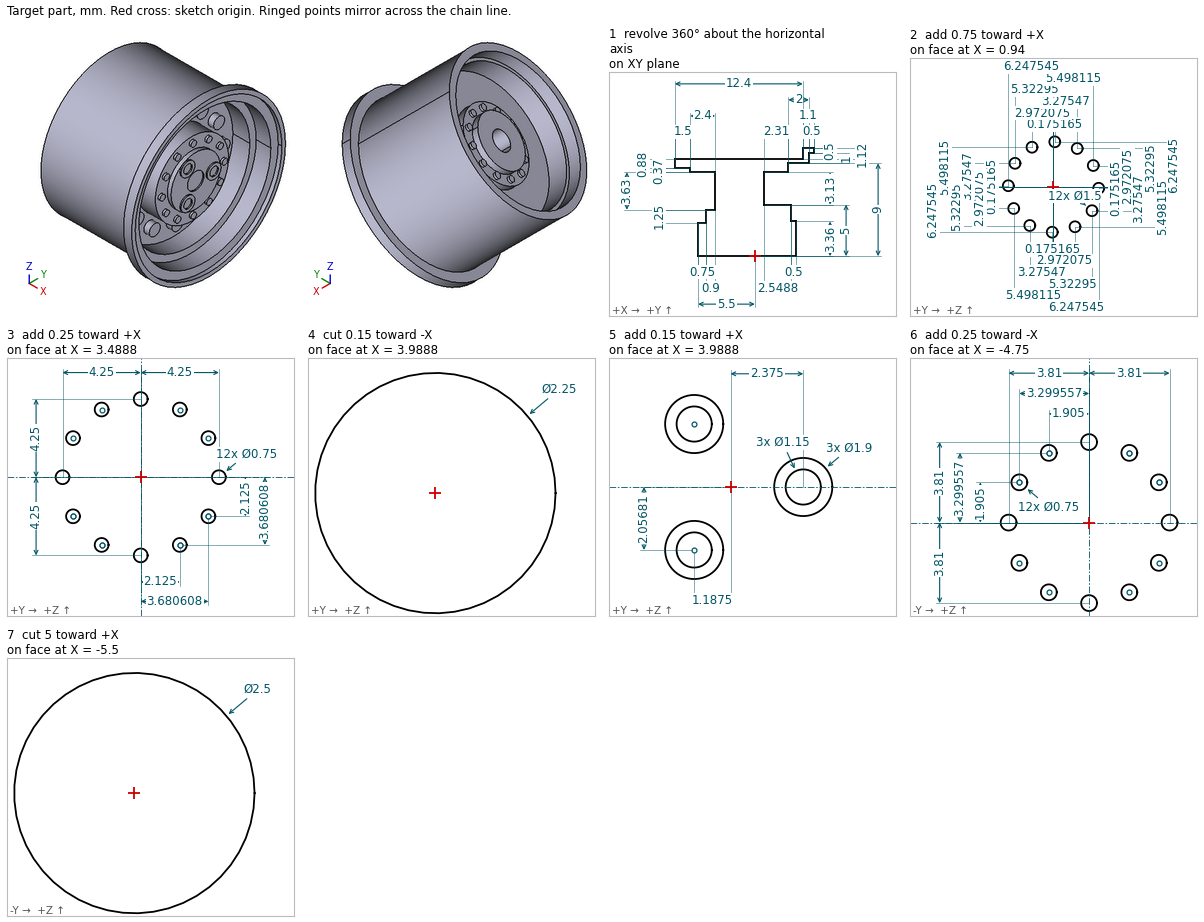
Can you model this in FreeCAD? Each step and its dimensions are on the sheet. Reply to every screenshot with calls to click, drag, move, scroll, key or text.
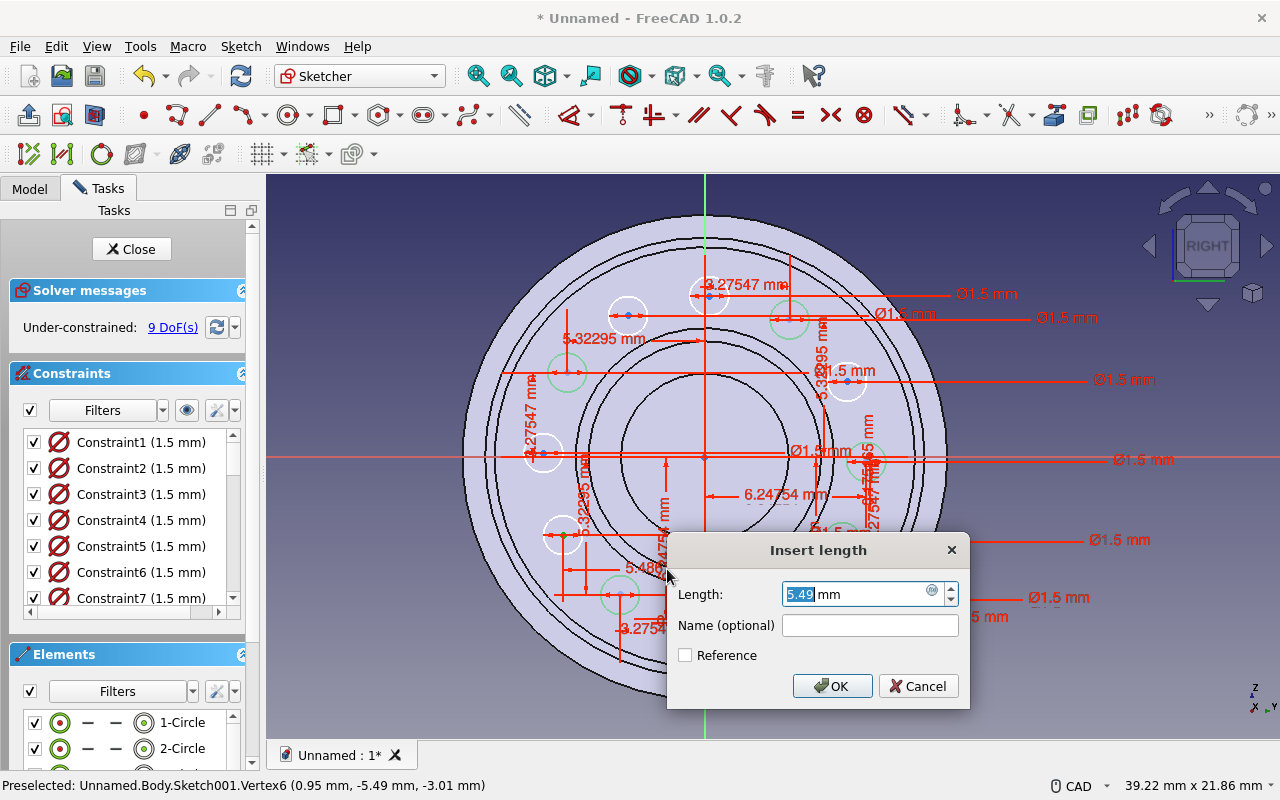
text(5.498115)
key(Return)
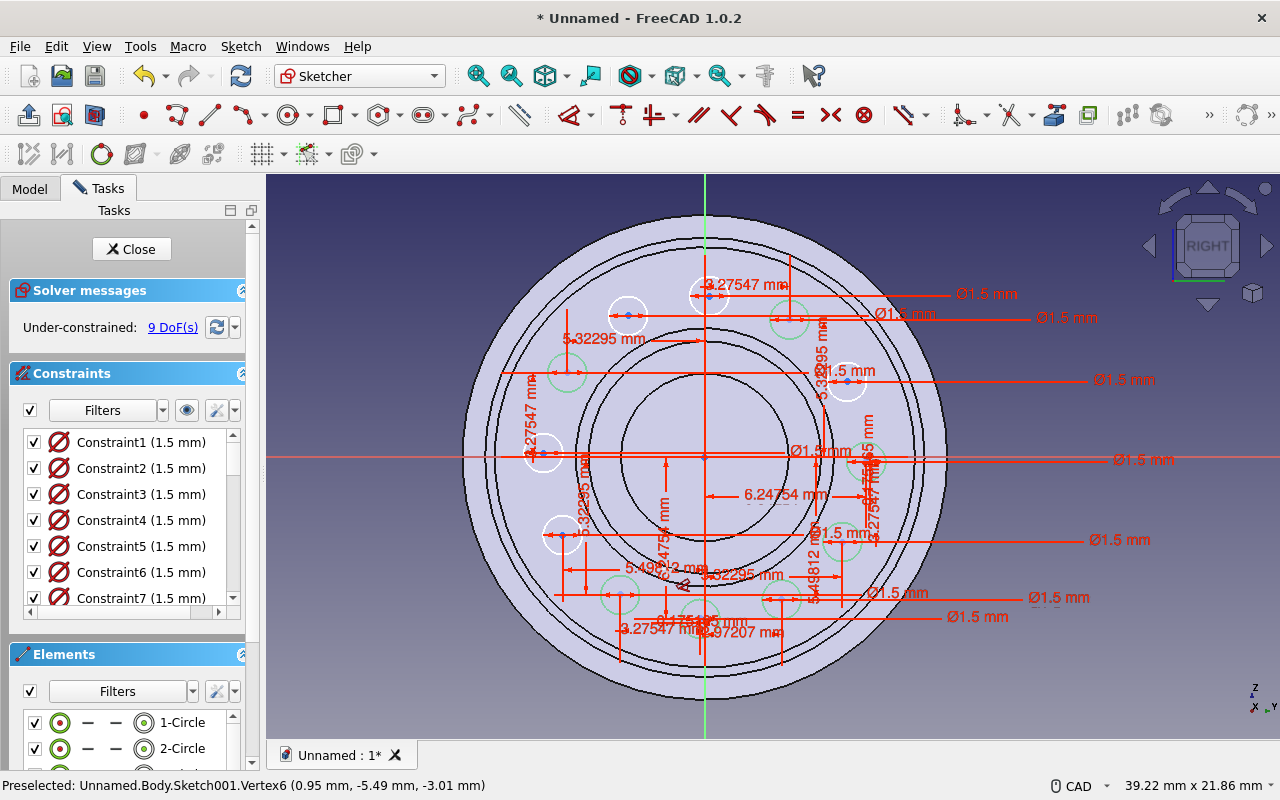
click(563, 535)
click(529, 523)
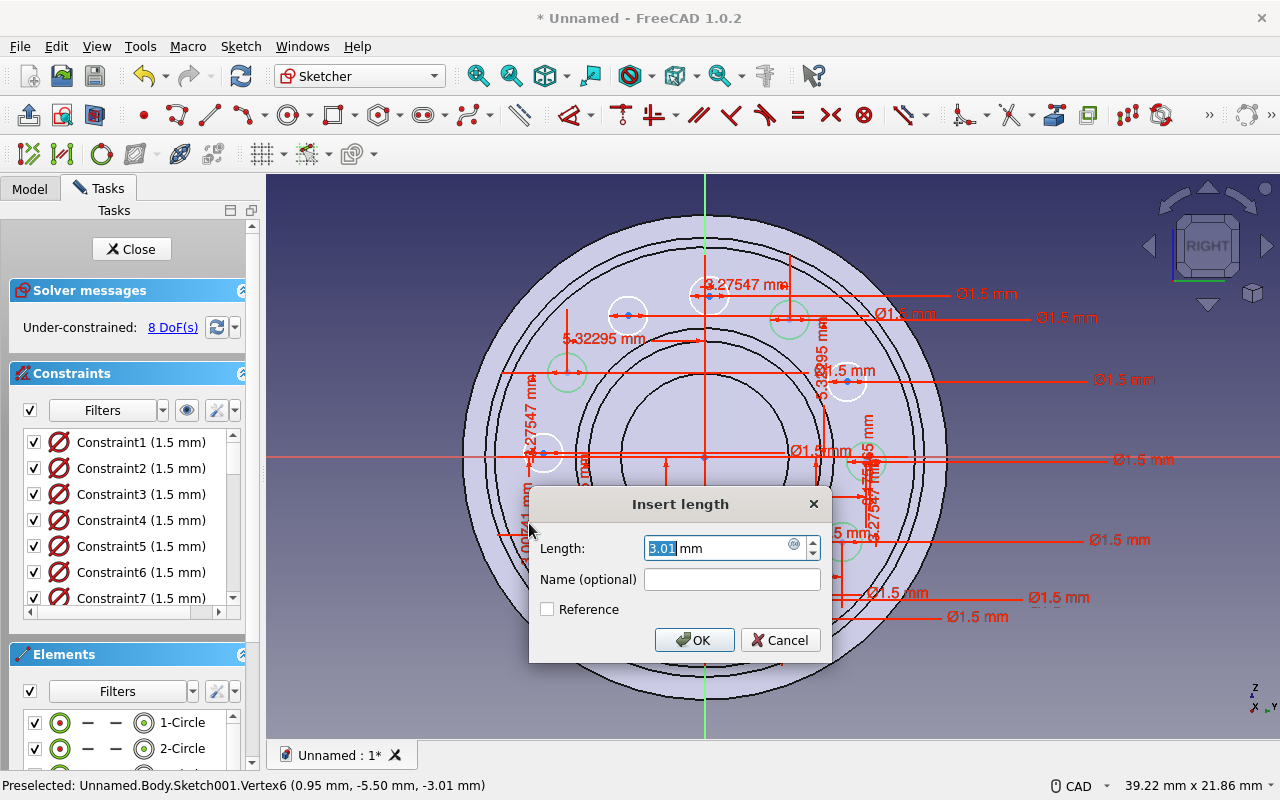
text(2.972075)
key(Return)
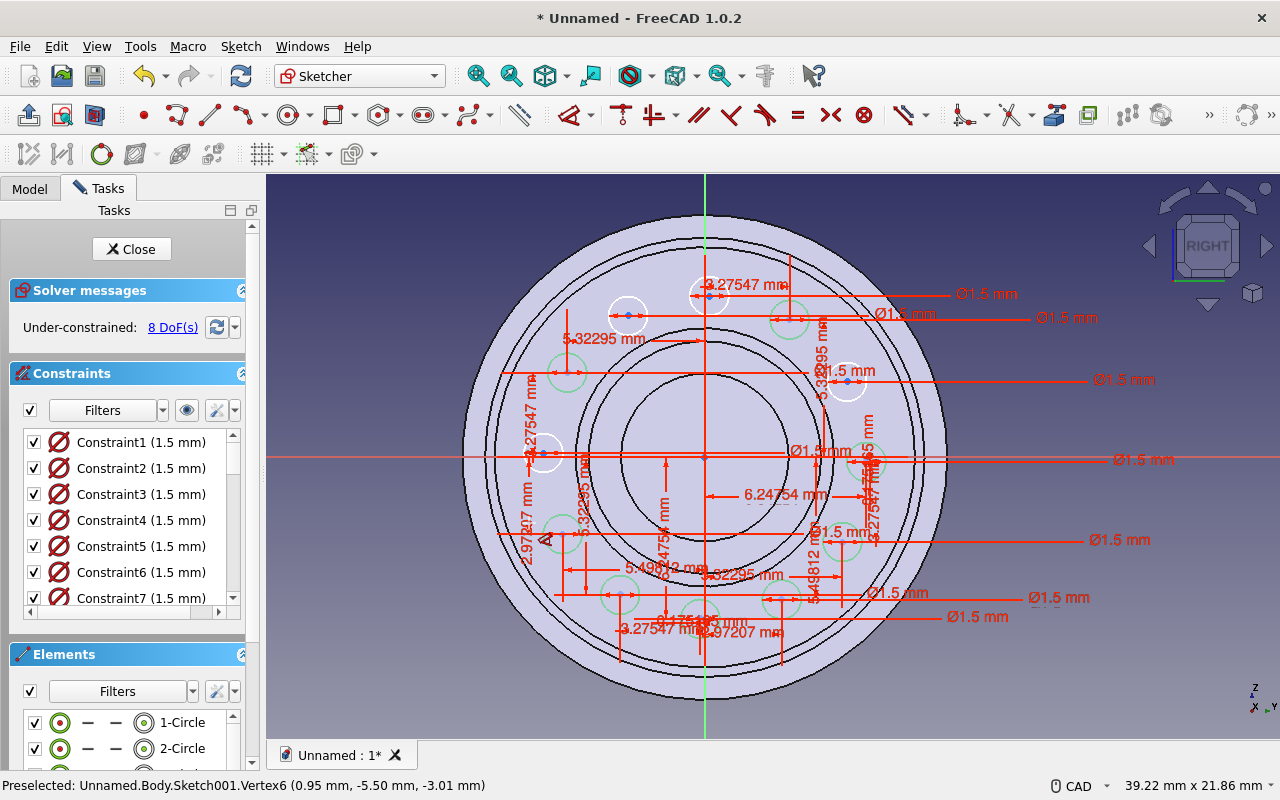
click(543, 453)
click(624, 419)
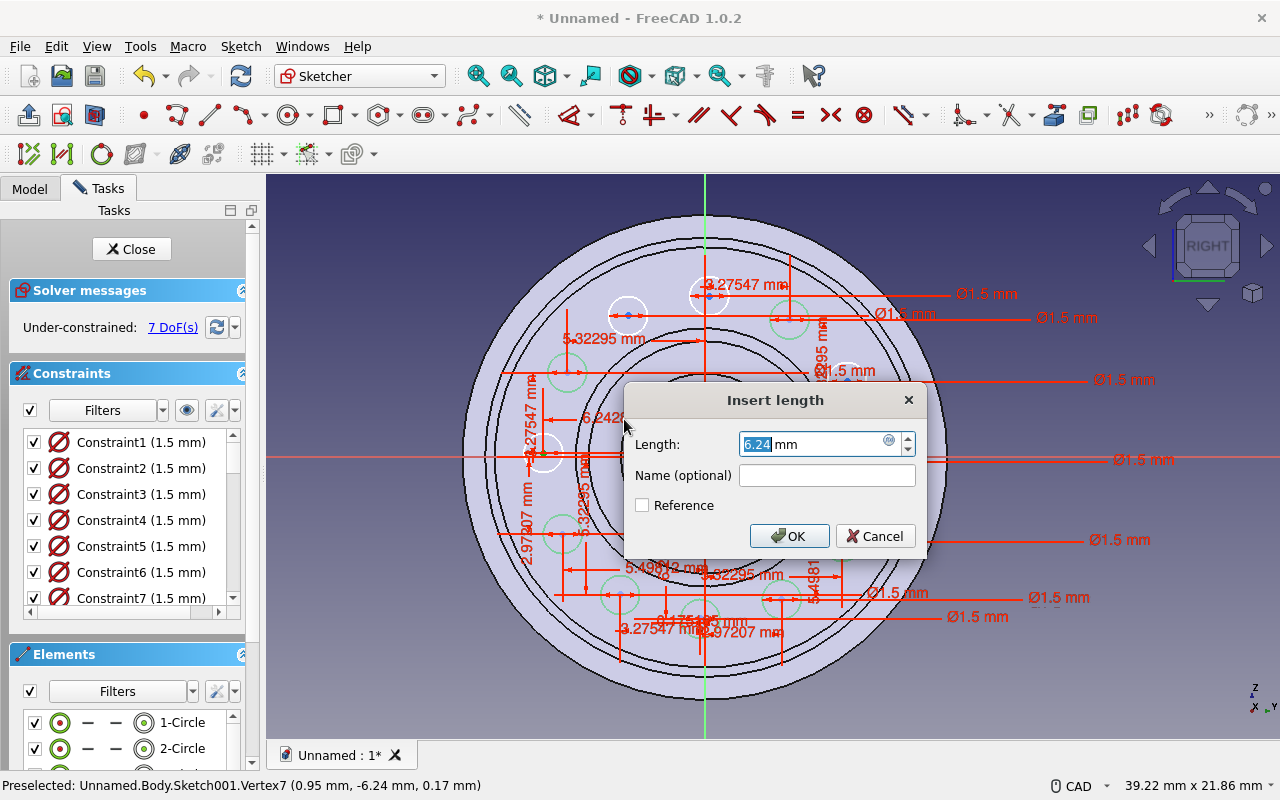
text(6.247545)
key(Return)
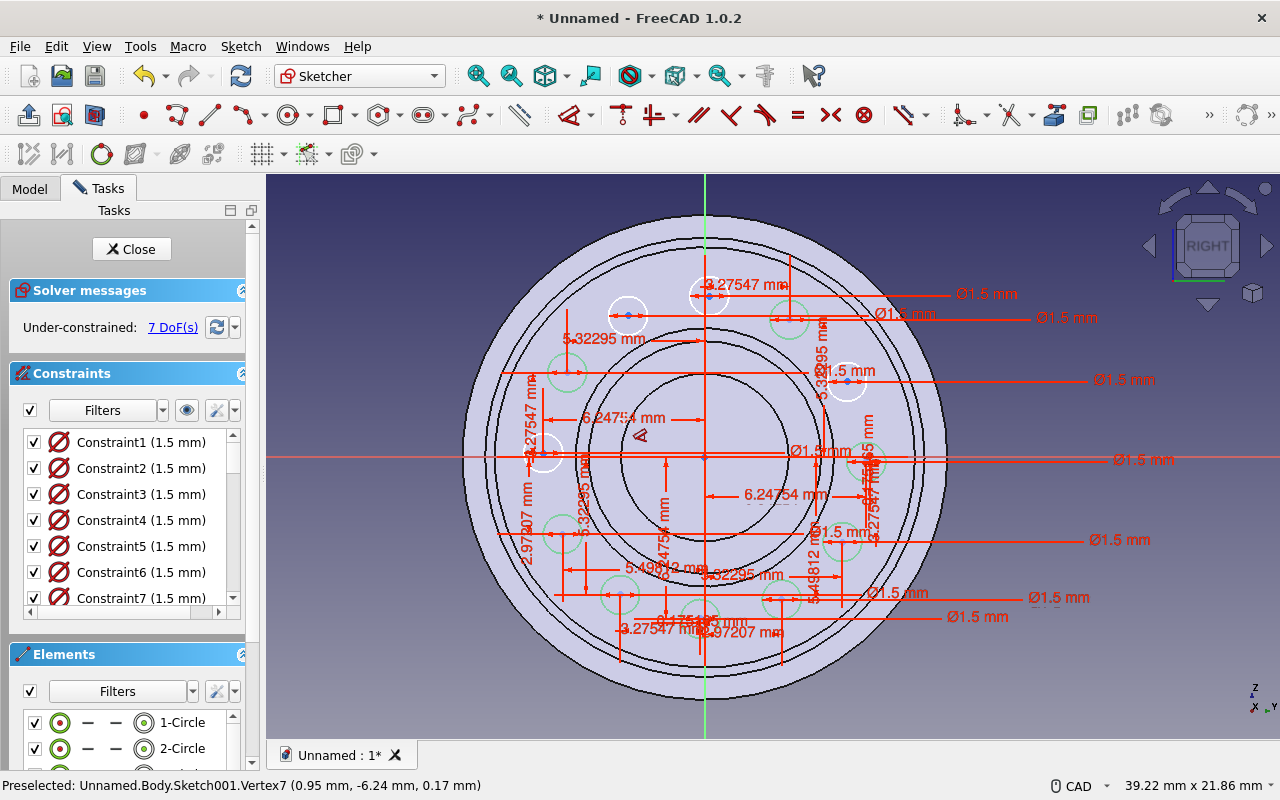
scroll(543, 453, up, 11)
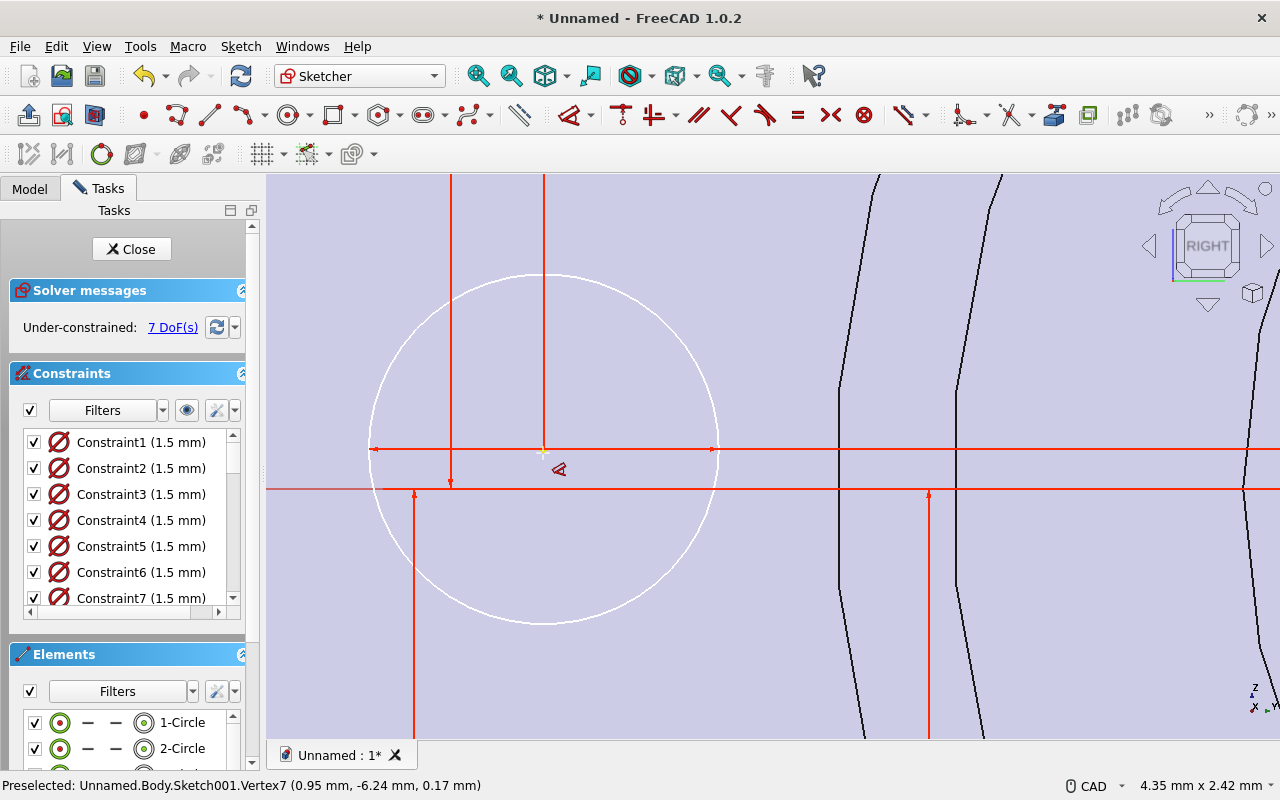
click(544, 449)
click(510, 469)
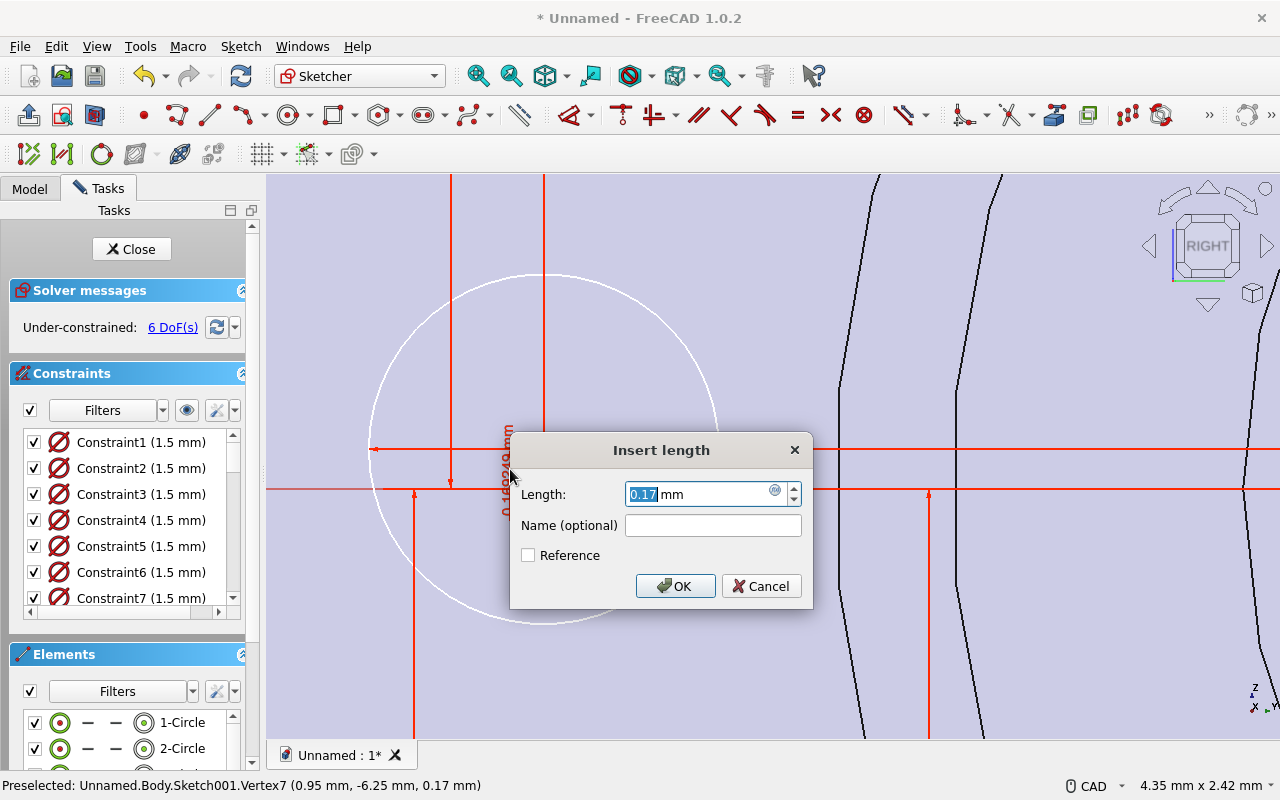
text(0.175165)
key(Return)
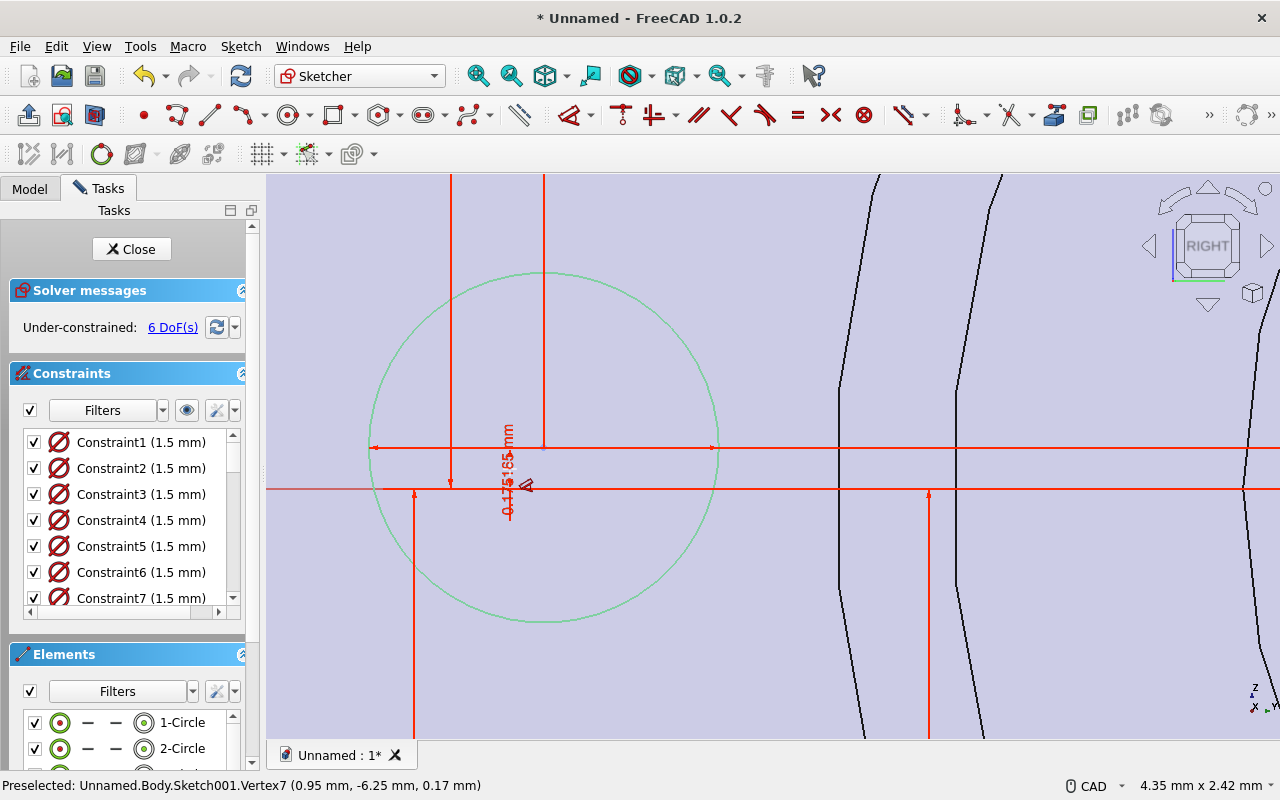
scroll(543, 452, down, 11)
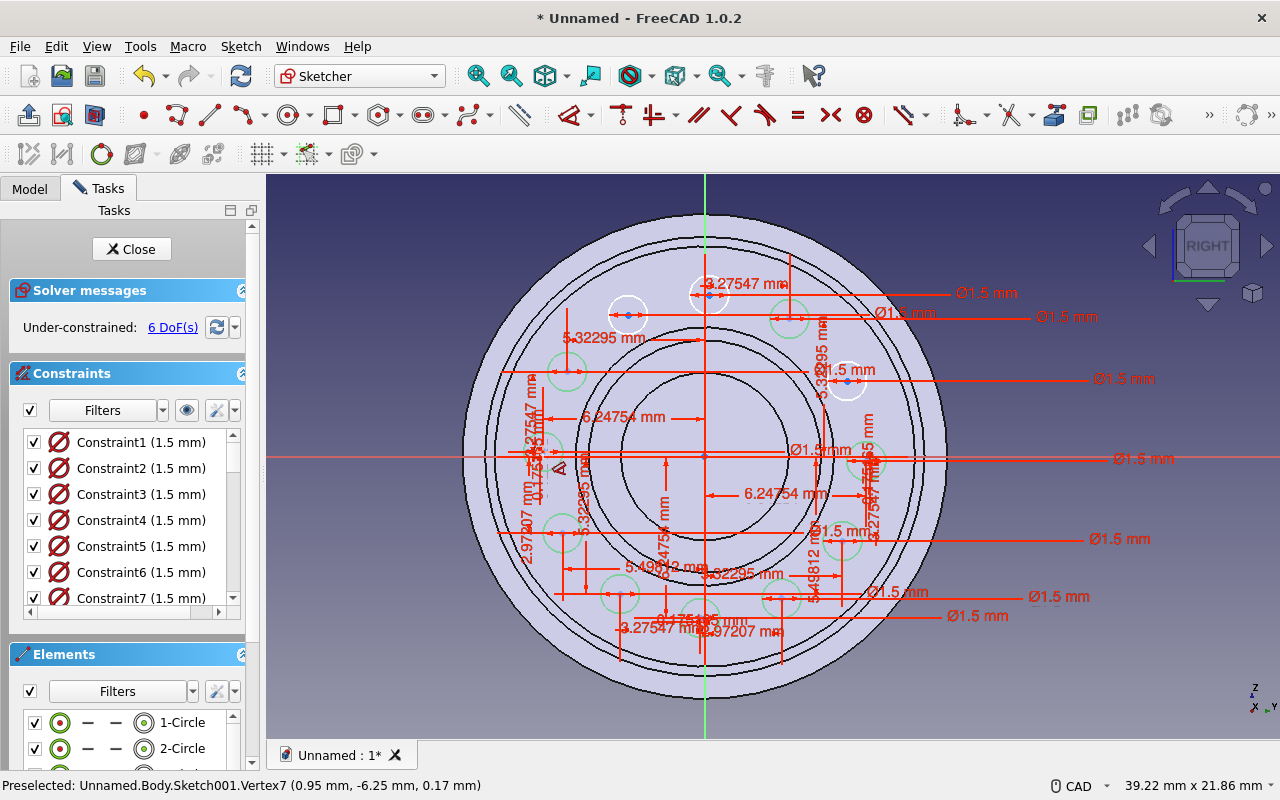
click(628, 315)
click(666, 281)